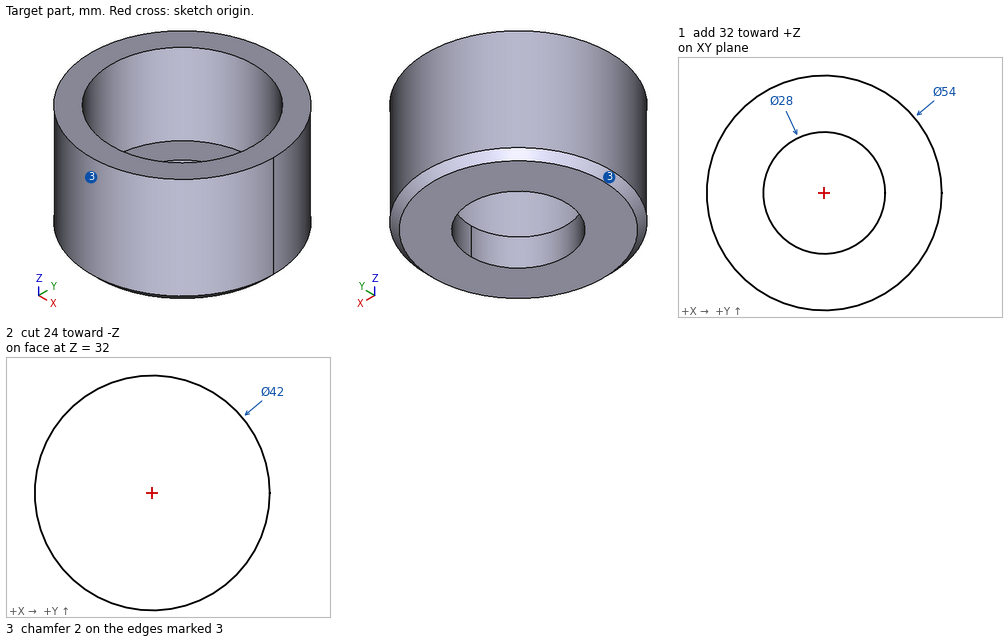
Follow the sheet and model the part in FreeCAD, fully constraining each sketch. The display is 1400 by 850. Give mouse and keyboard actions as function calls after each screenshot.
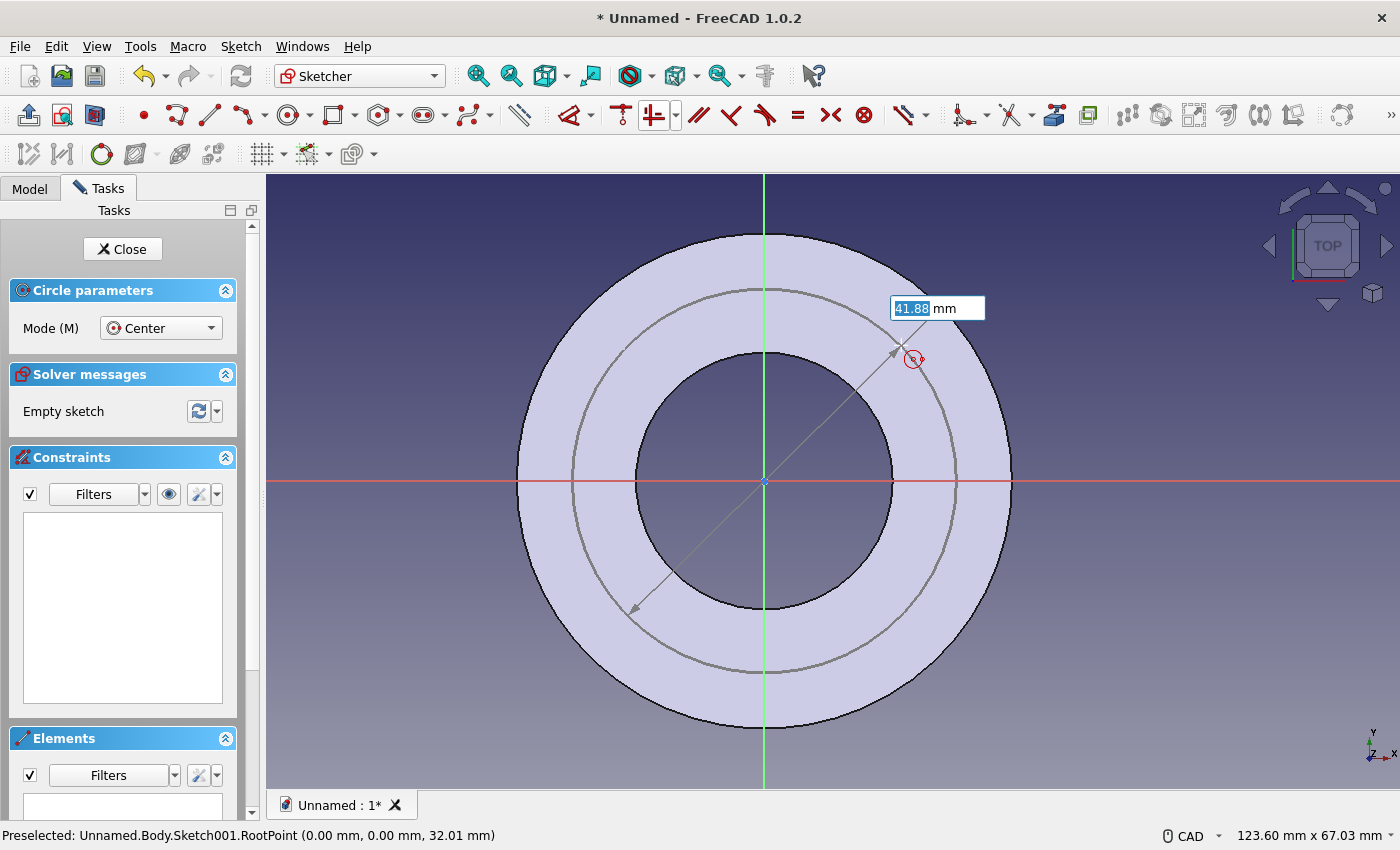
text(42)
key(Return)
key(Escape)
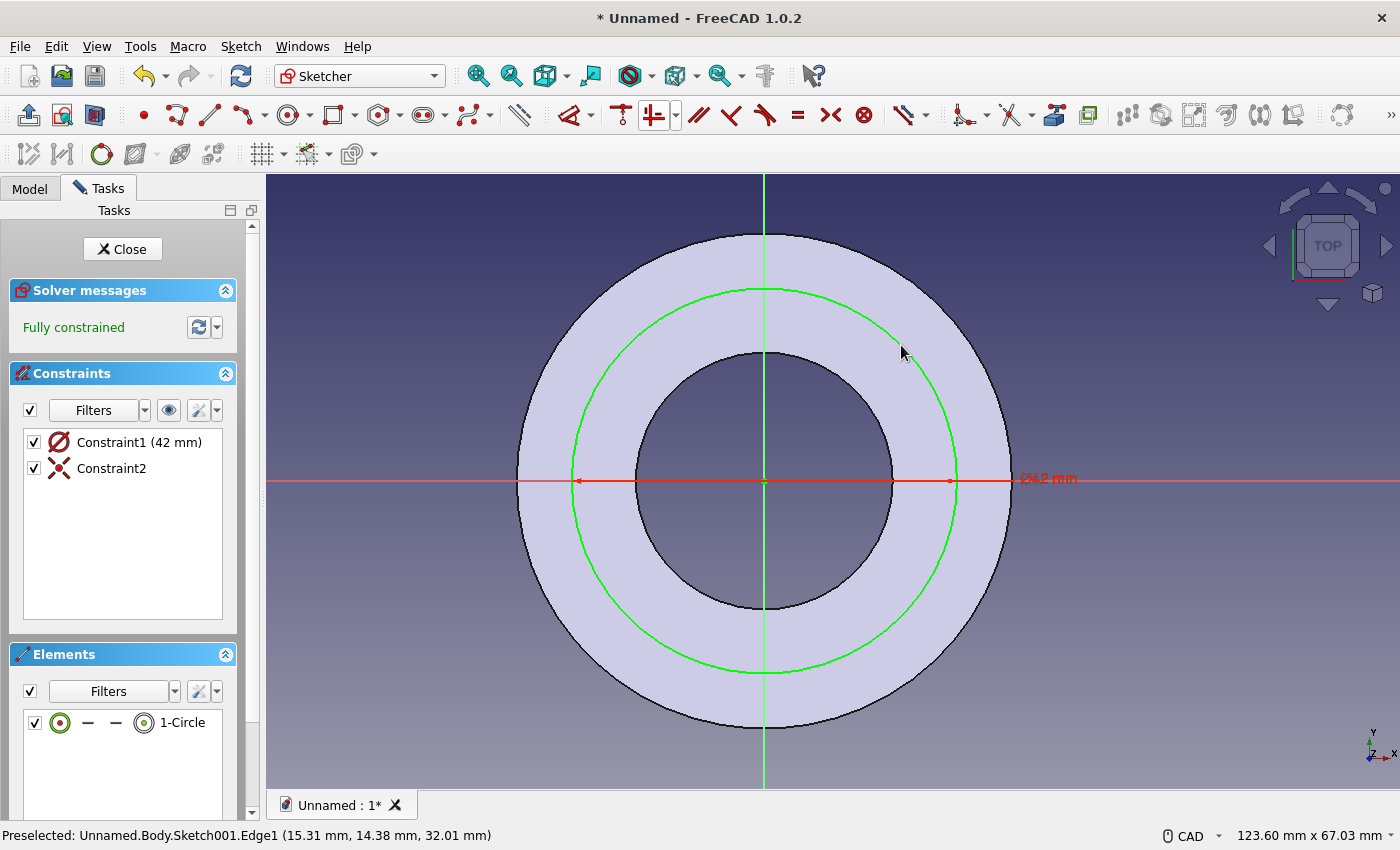
click(123, 249)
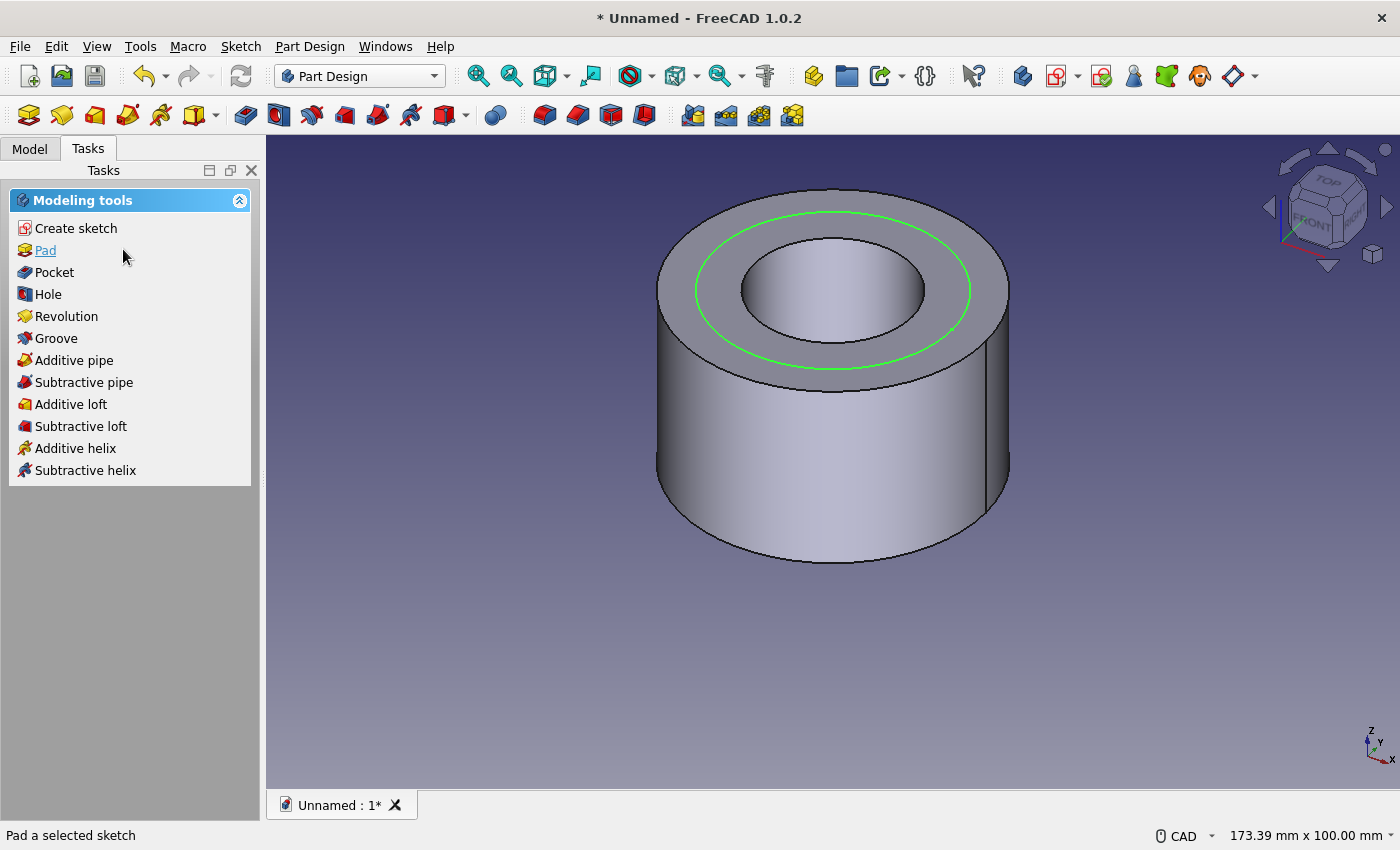
click(246, 116)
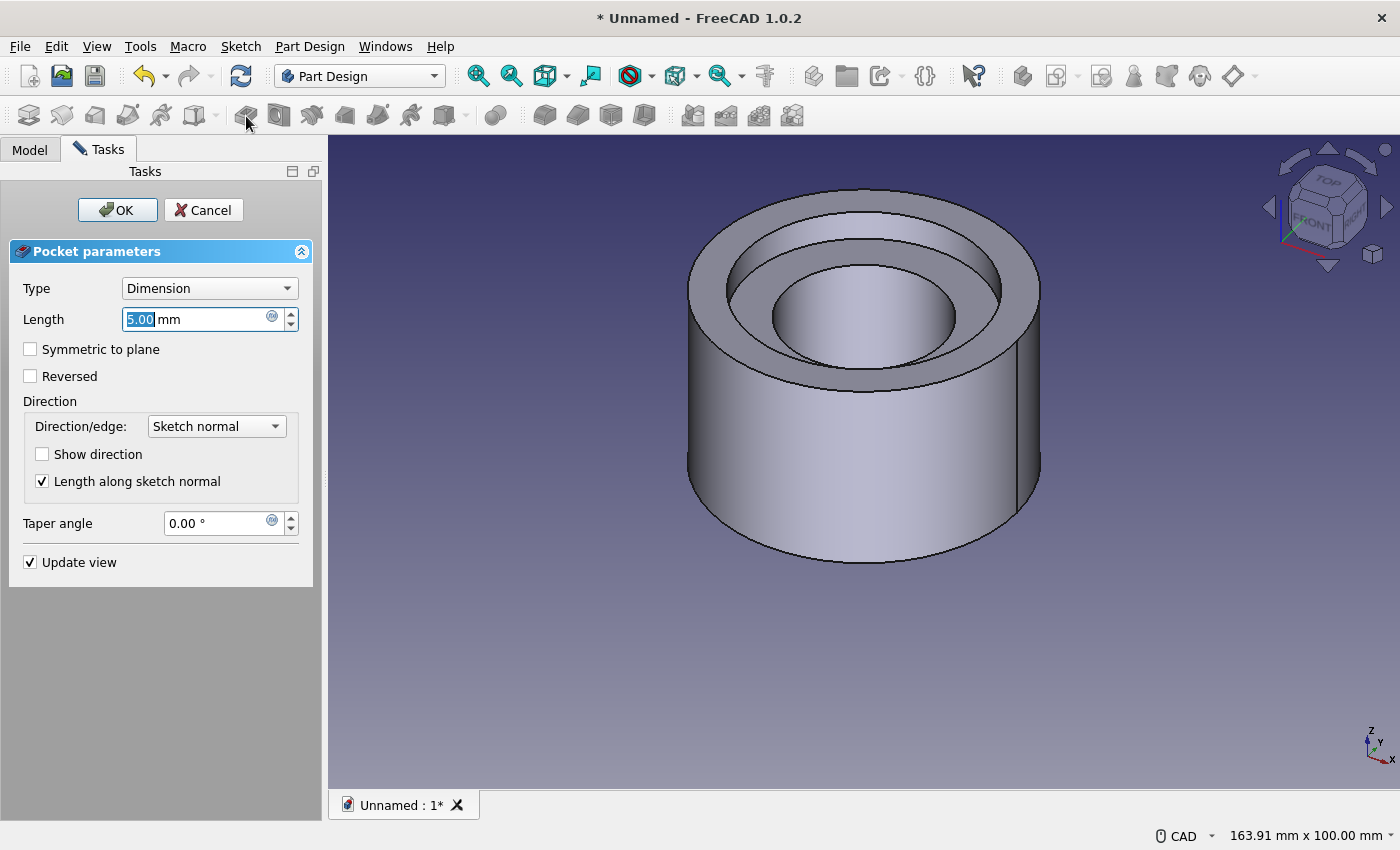
text(24)
key(Tab)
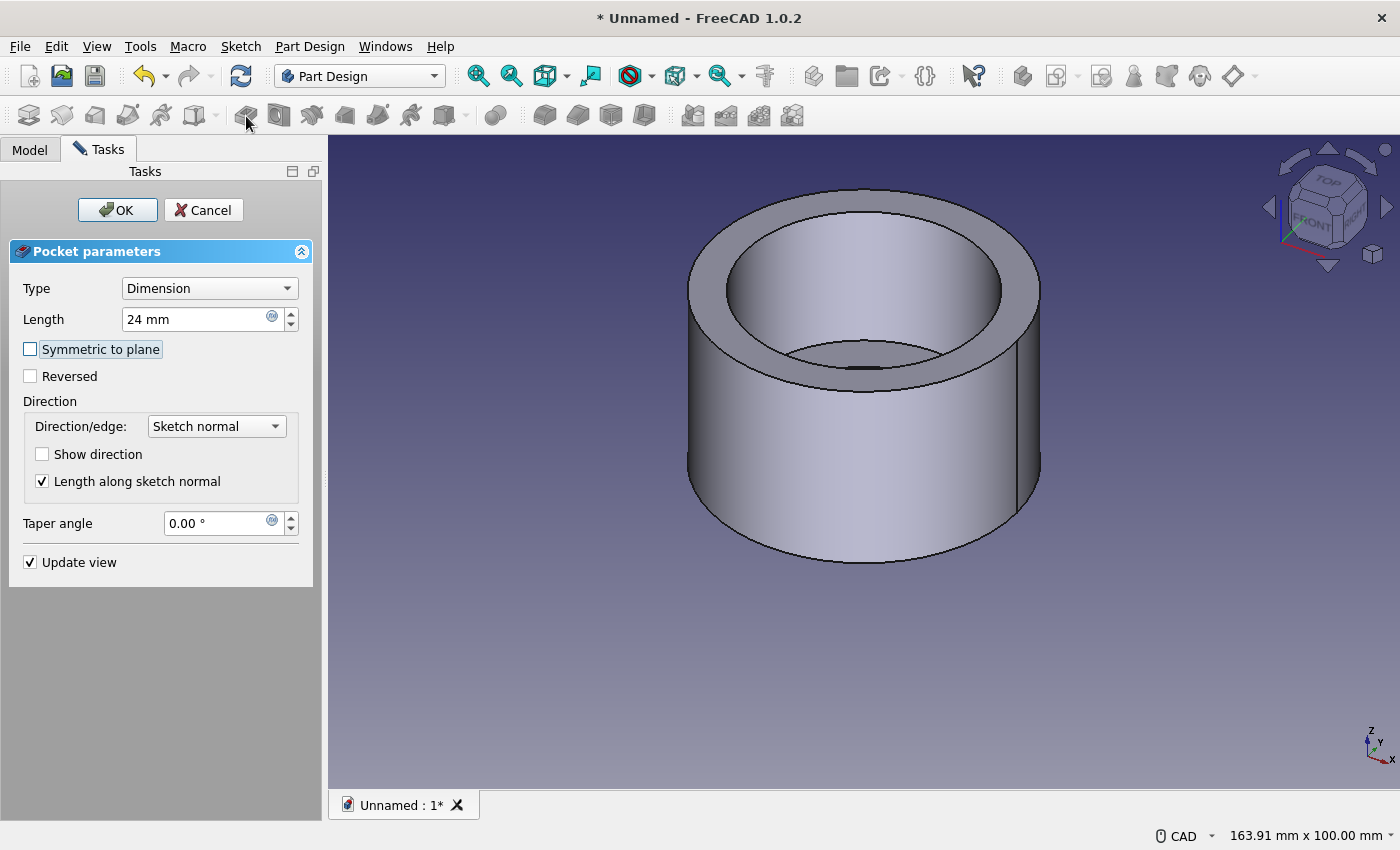
click(118, 210)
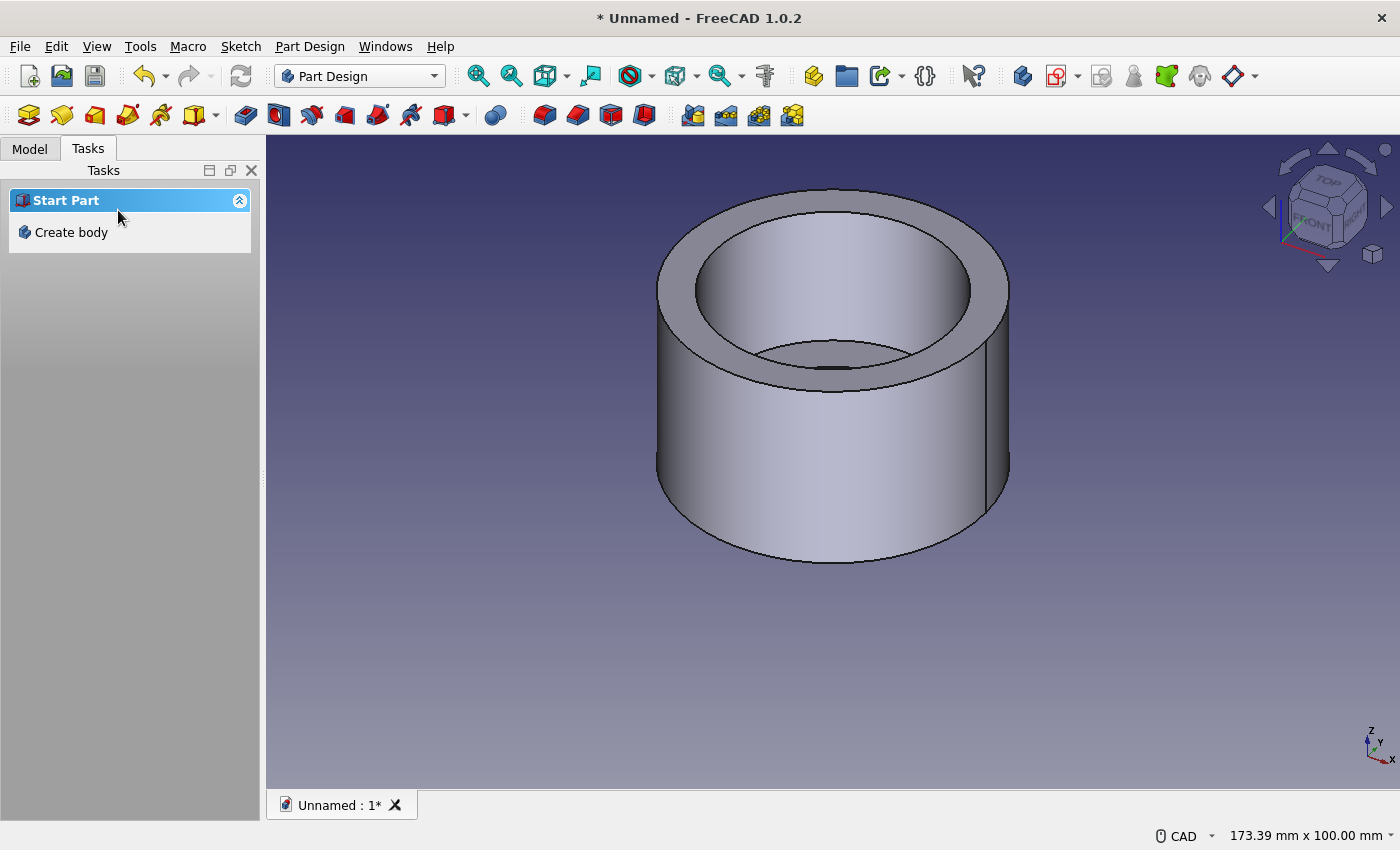
key(0)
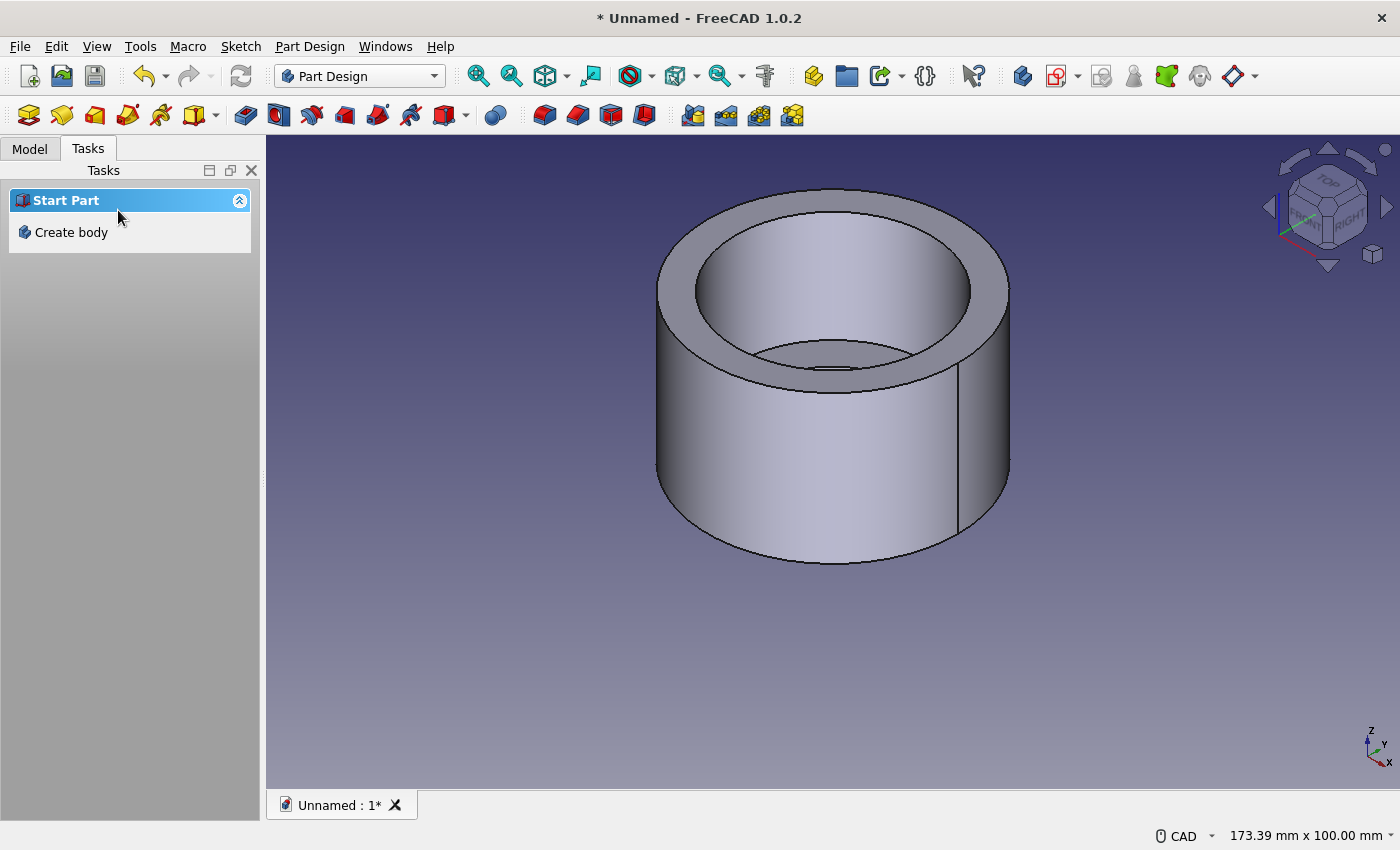
key(2)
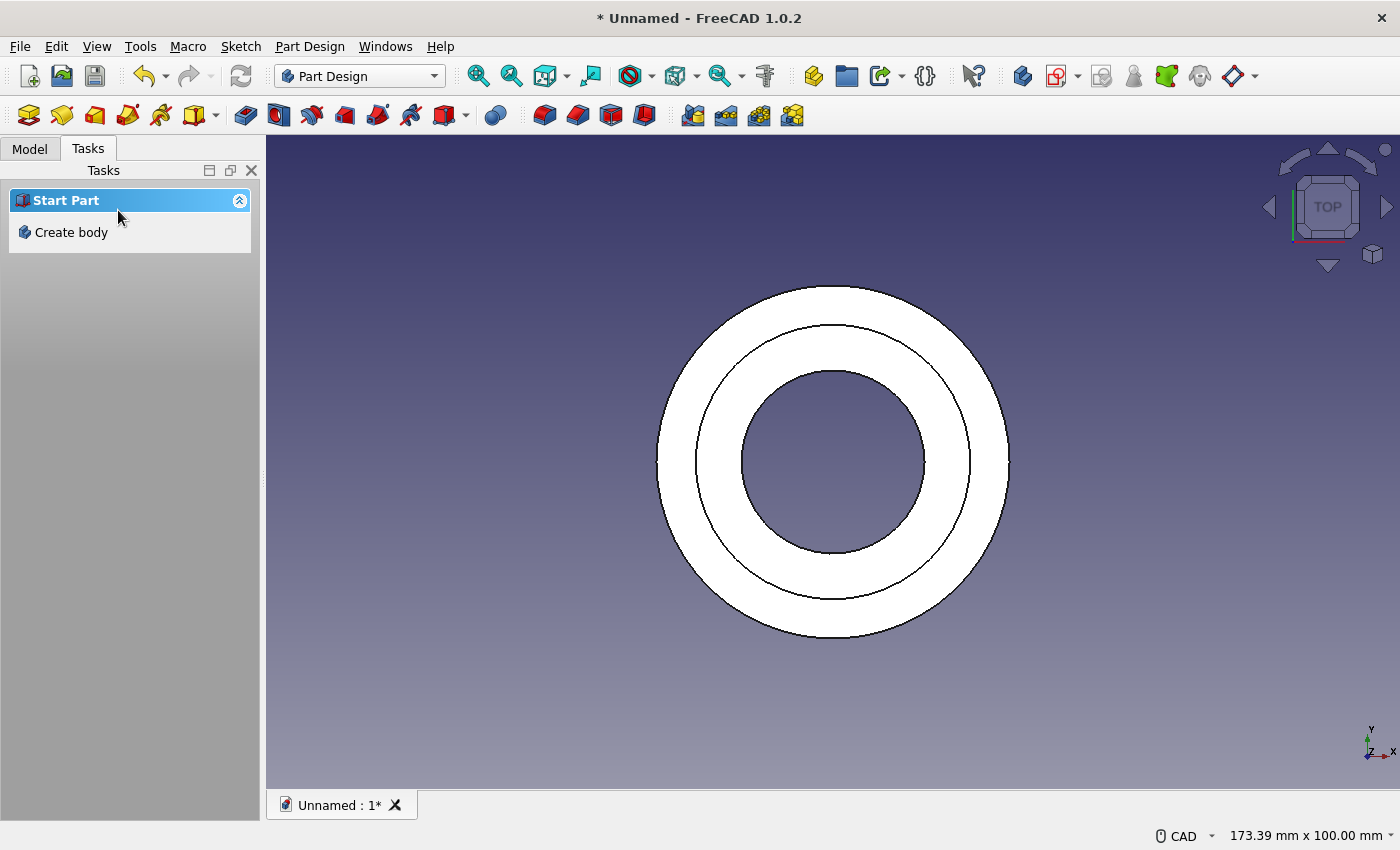
key(1)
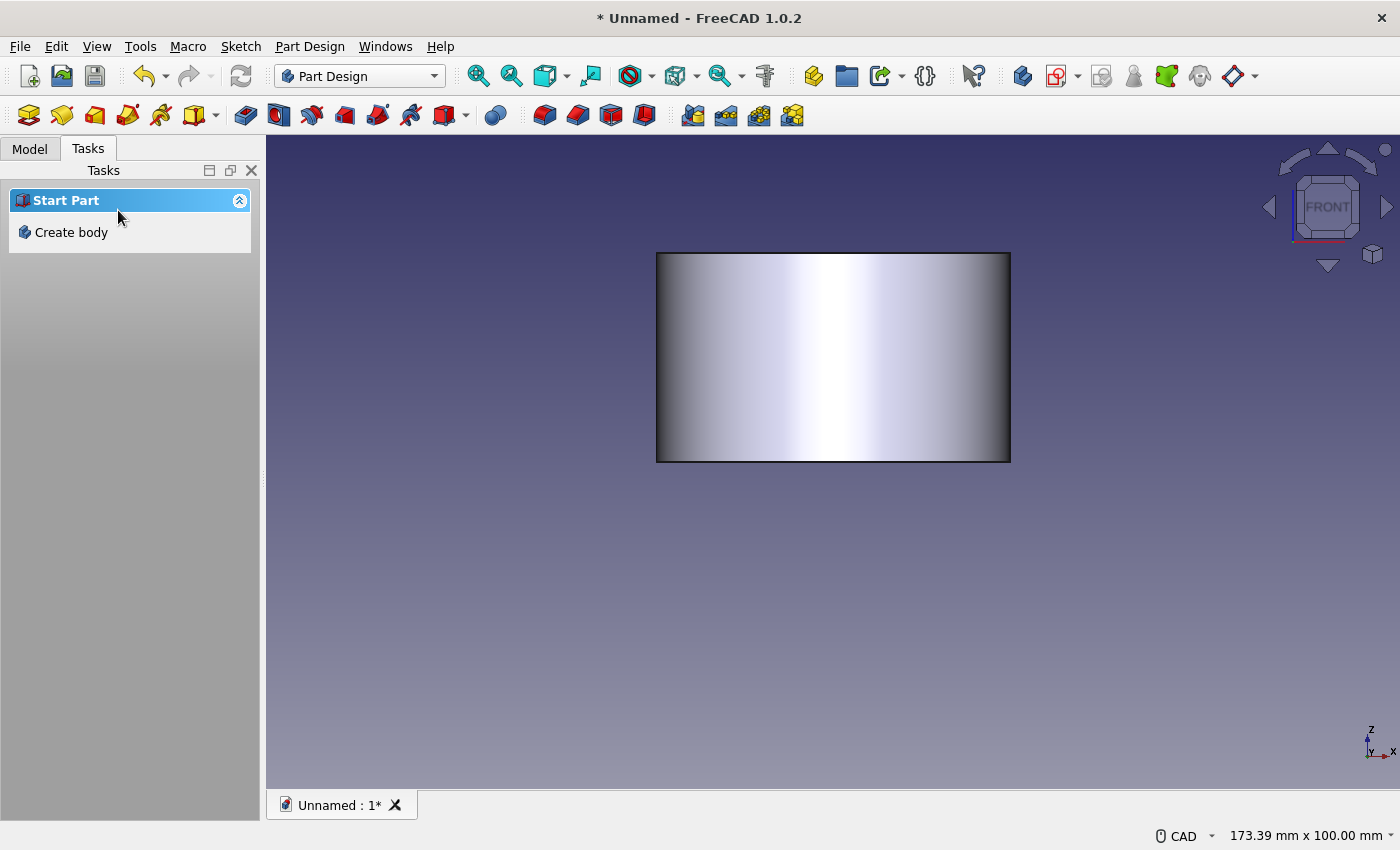
key(v)
key(f)